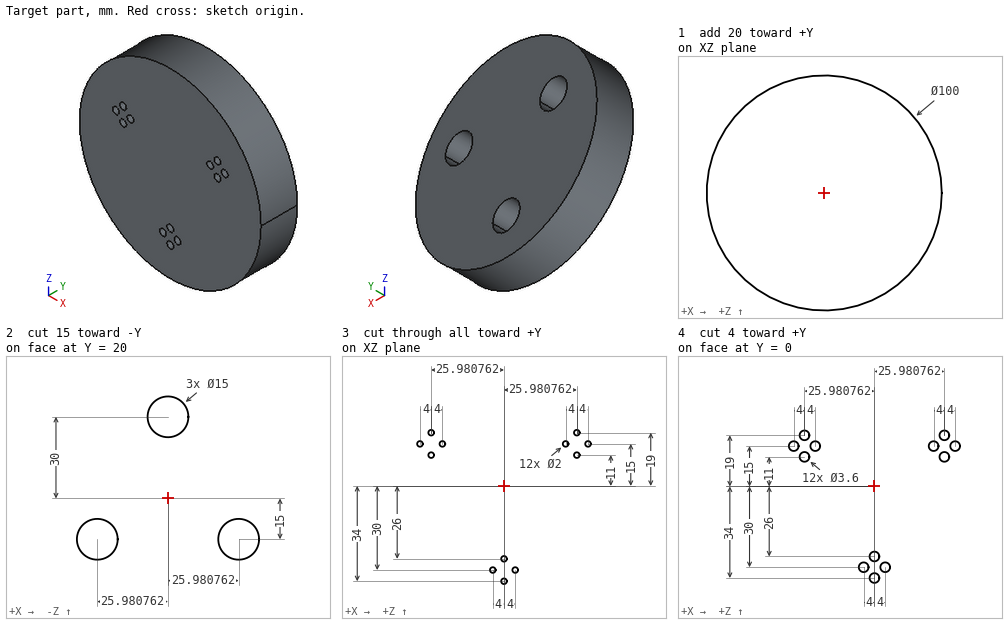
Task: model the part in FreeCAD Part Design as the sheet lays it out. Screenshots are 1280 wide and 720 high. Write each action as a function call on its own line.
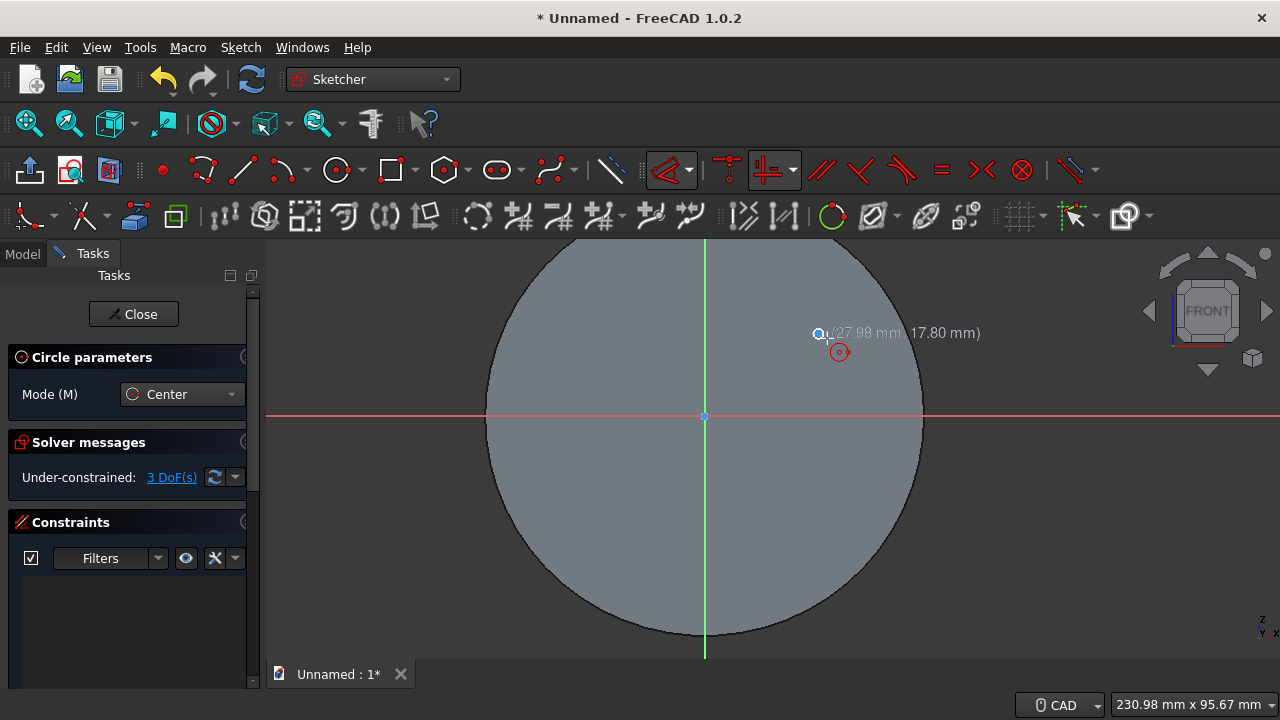
click(836, 351)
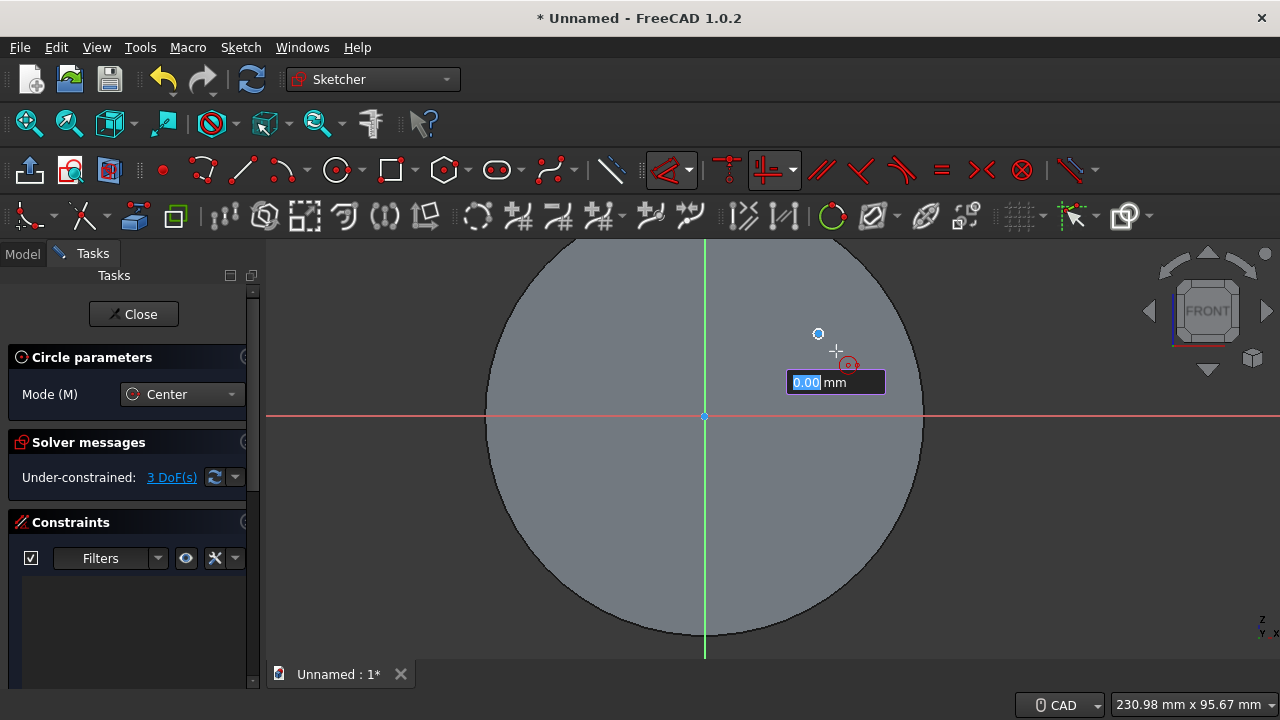
scroll(839, 348, up, 7)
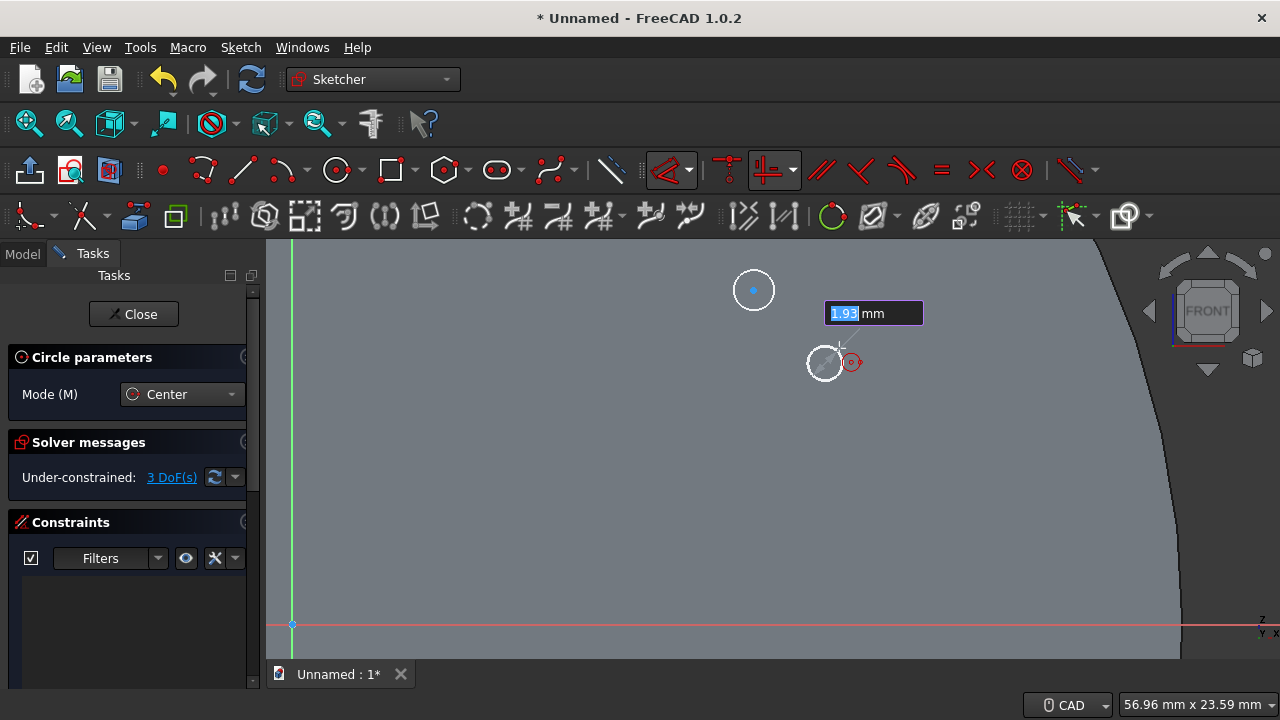
click(839, 345)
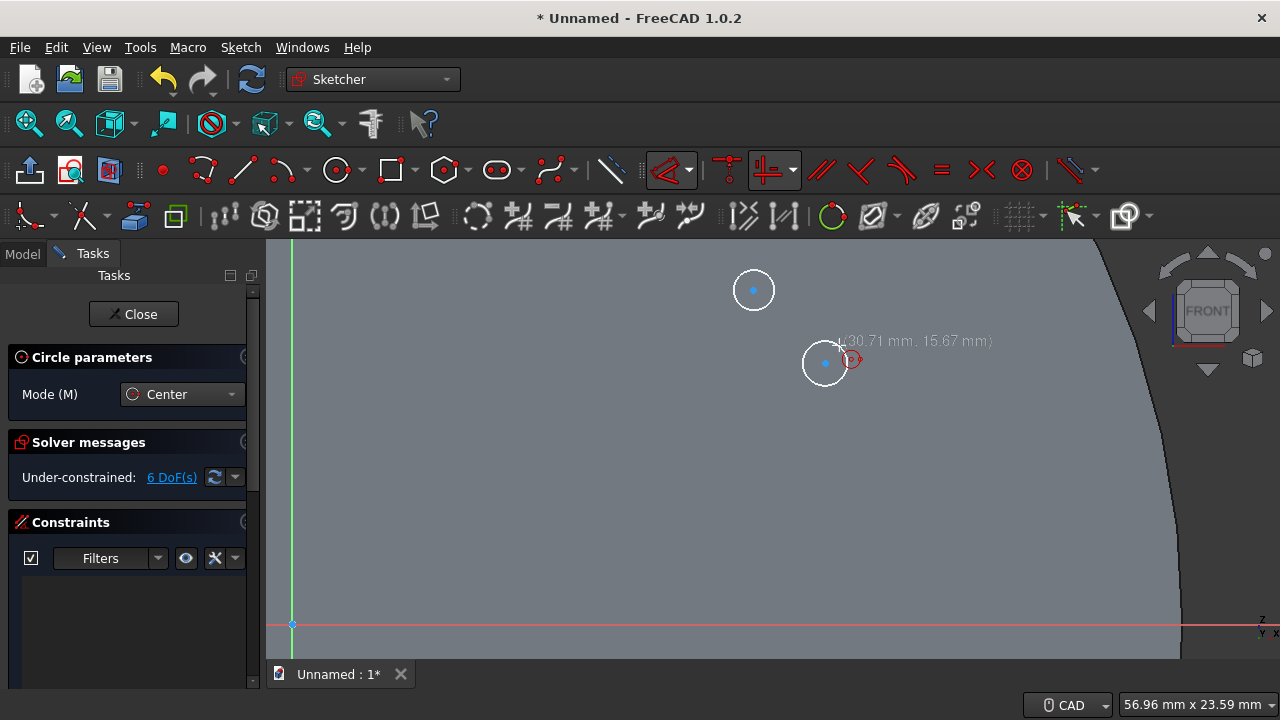
scroll(684, 358, up, 2)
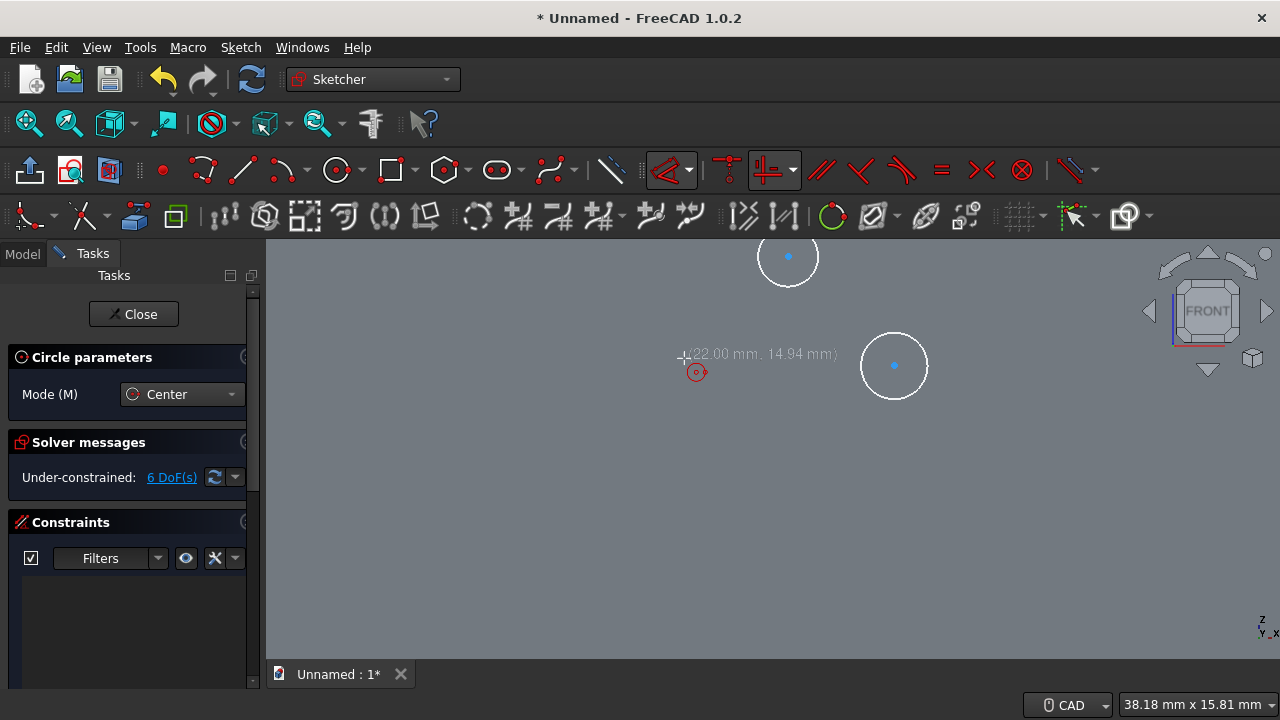
scroll(824, 349, down, 9)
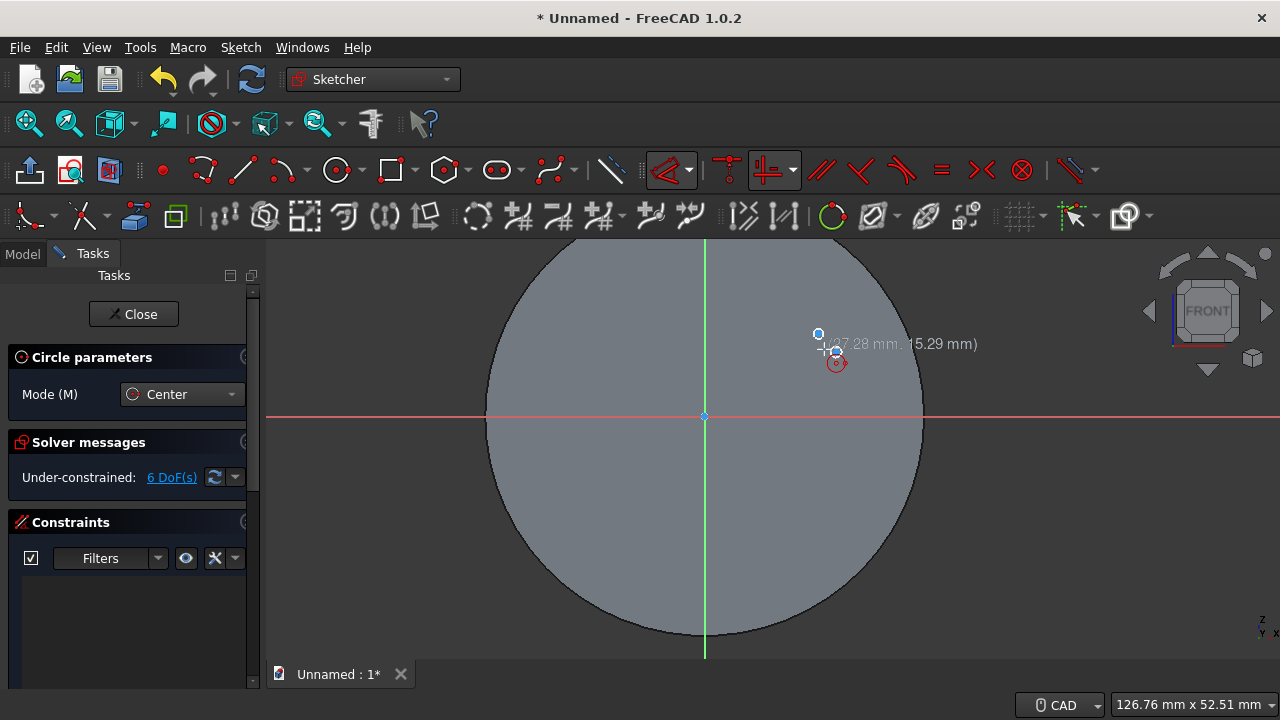
click(801, 351)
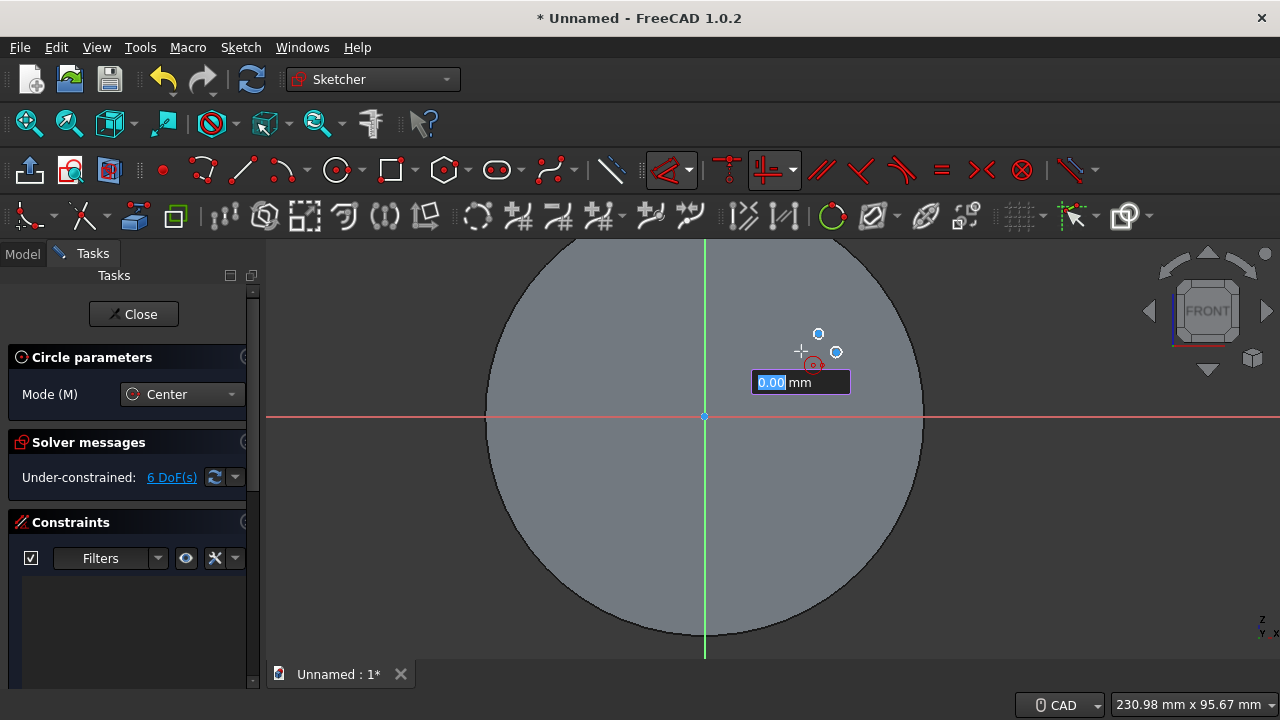
scroll(804, 348, up, 7)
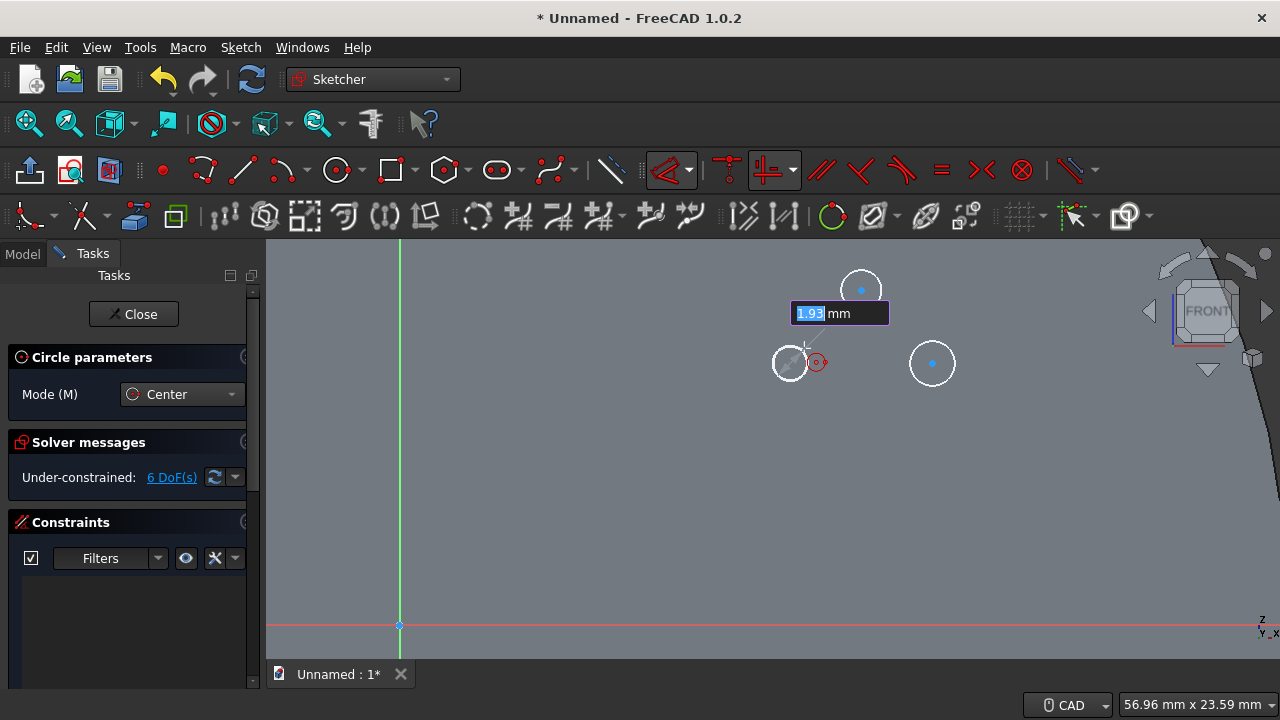
click(804, 345)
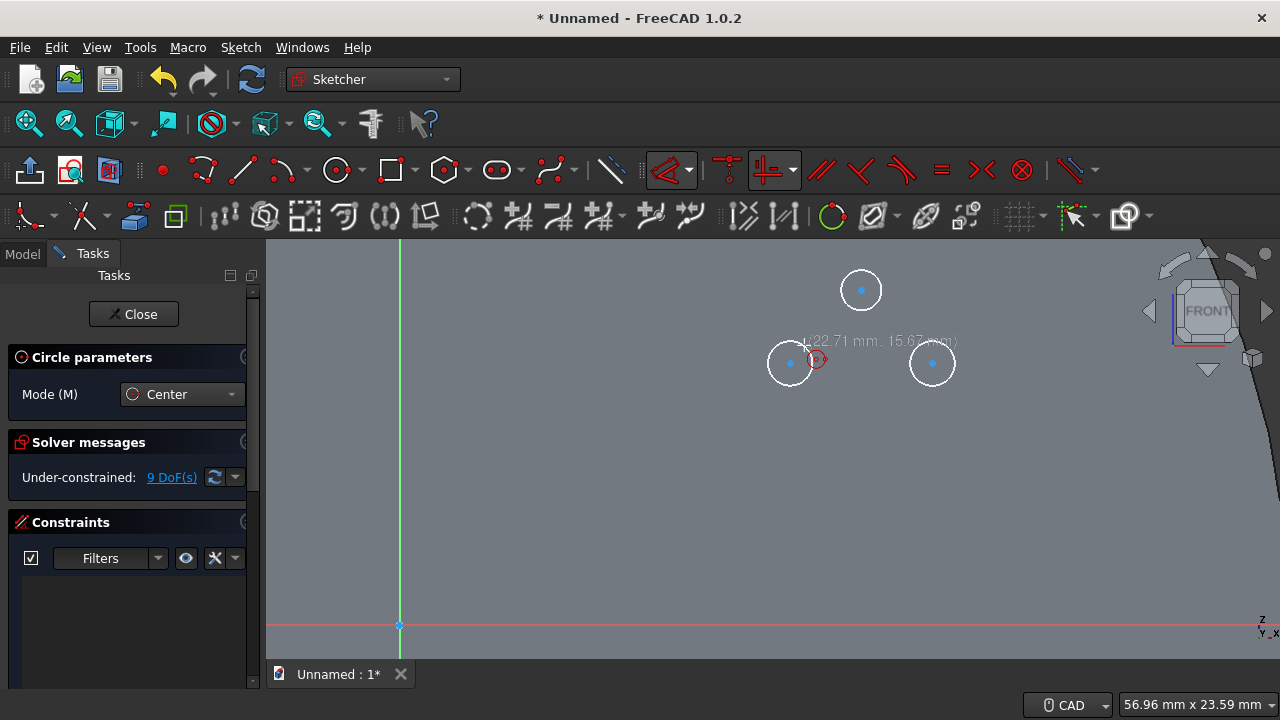
scroll(862, 429, up, 2)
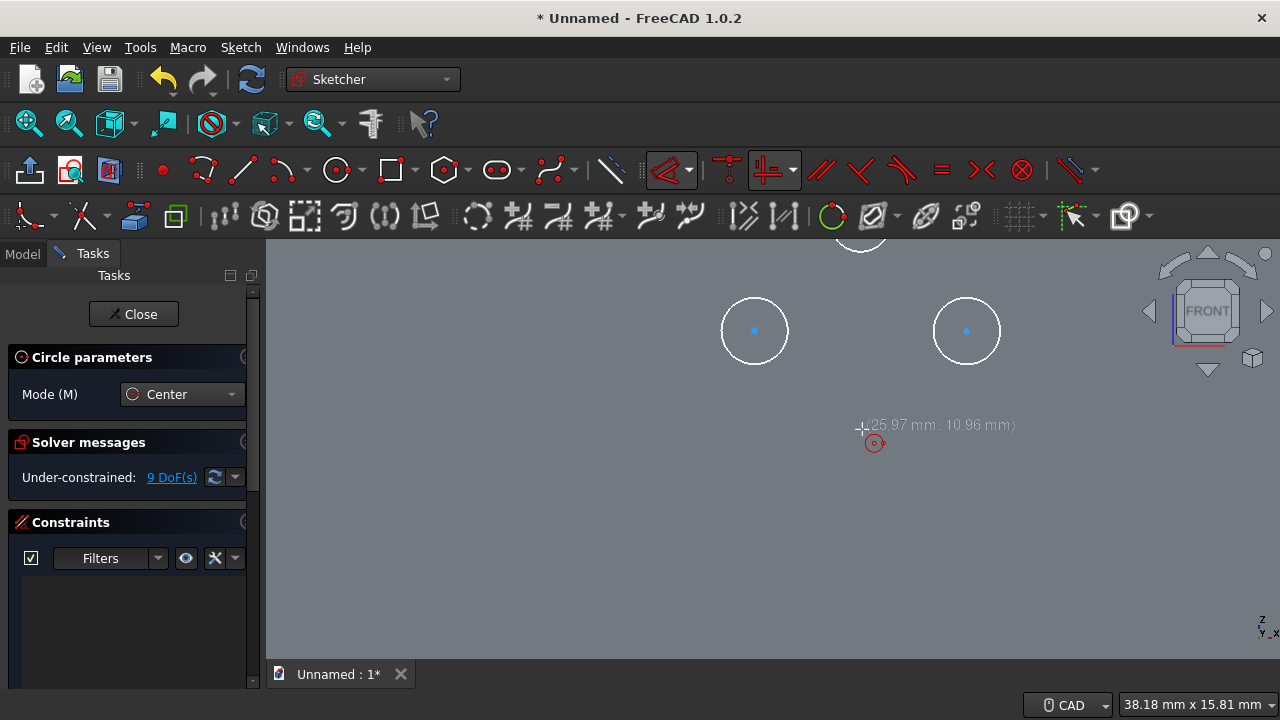
scroll(810, 356, down, 9)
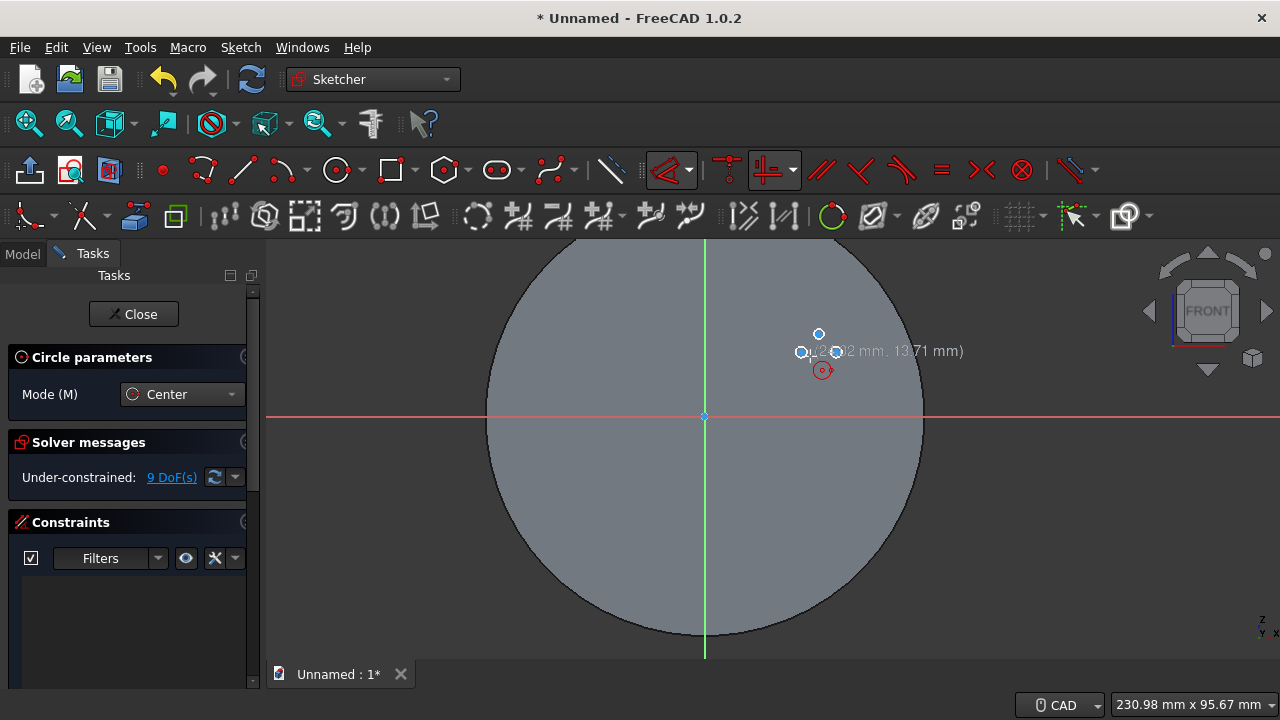
click(819, 368)